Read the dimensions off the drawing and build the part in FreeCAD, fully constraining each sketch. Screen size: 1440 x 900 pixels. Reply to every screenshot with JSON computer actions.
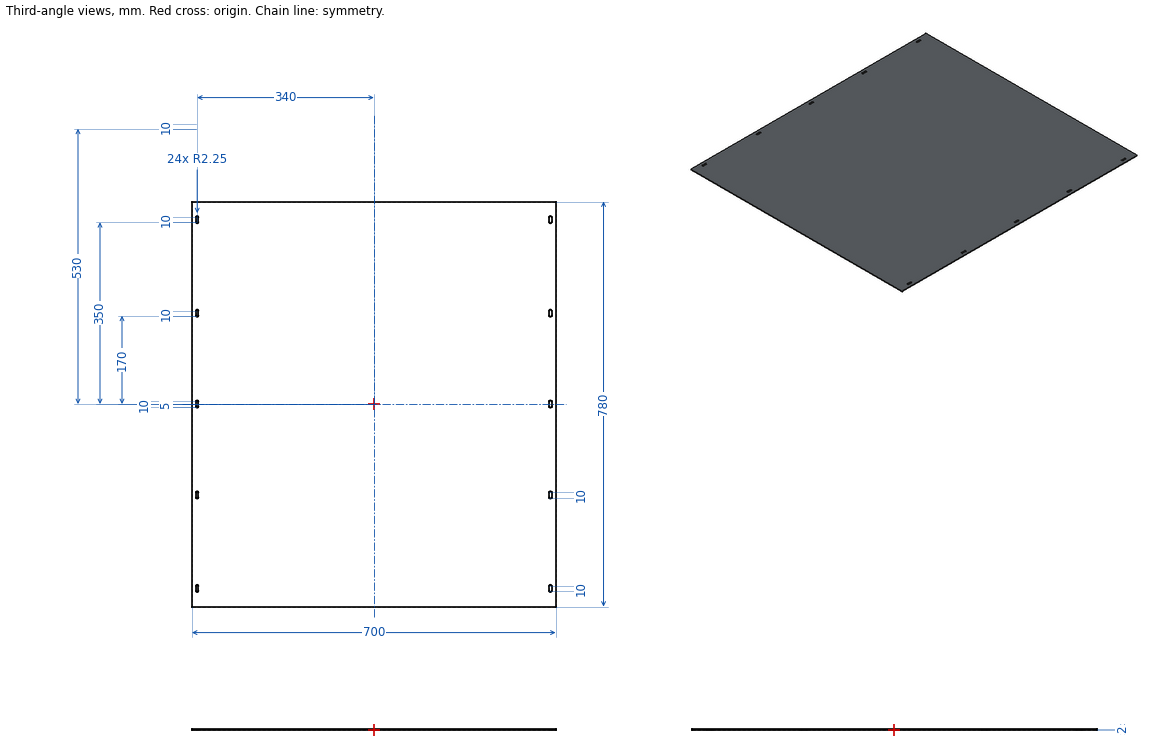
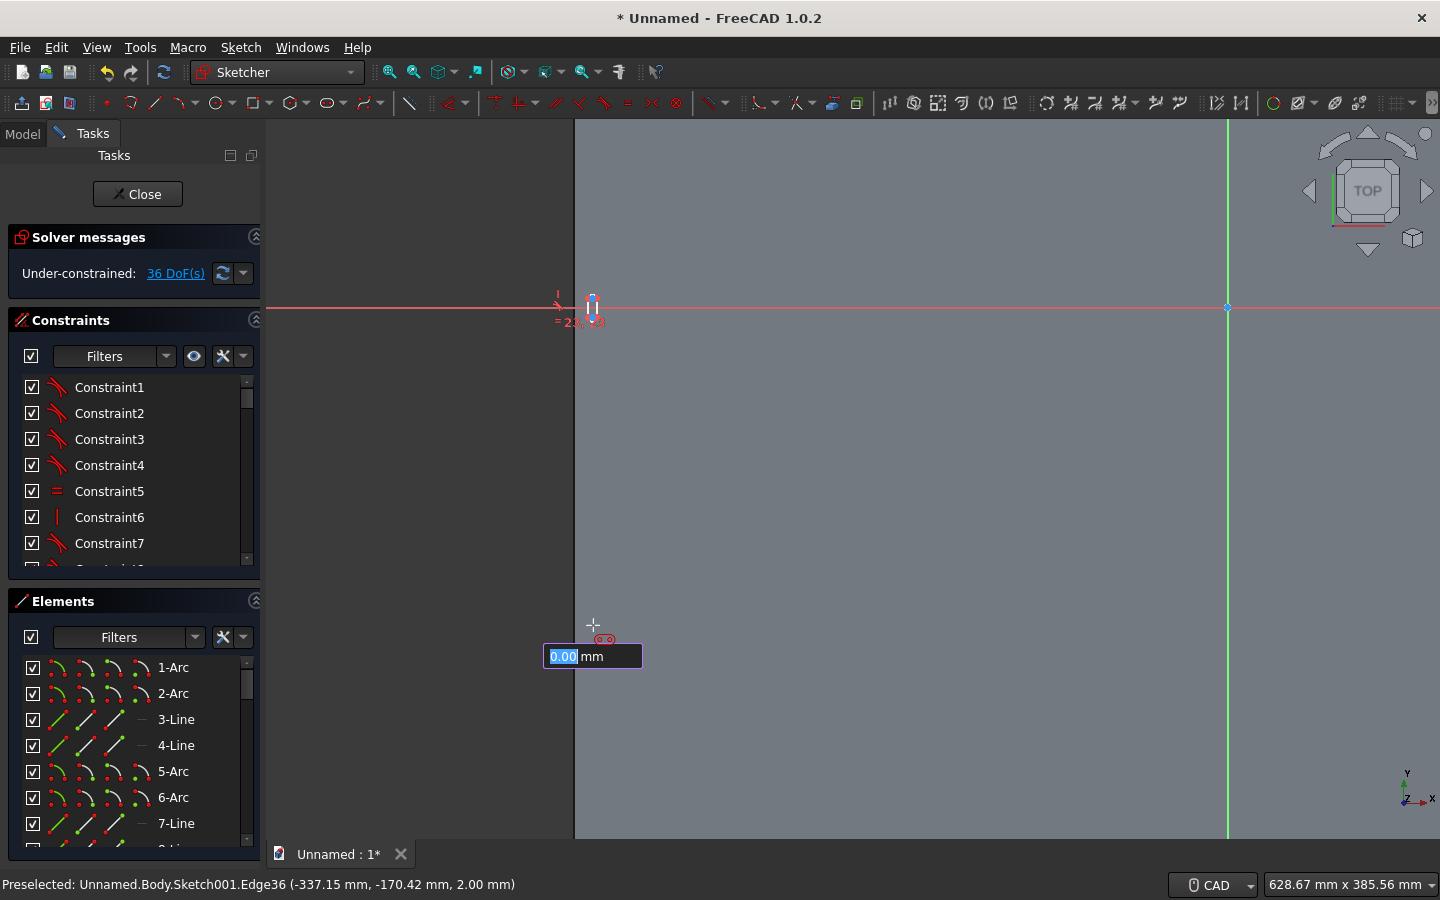
{"action": "scroll", "coordinate": [588, 634], "scroll_direction": "up", "scroll_amount": 7}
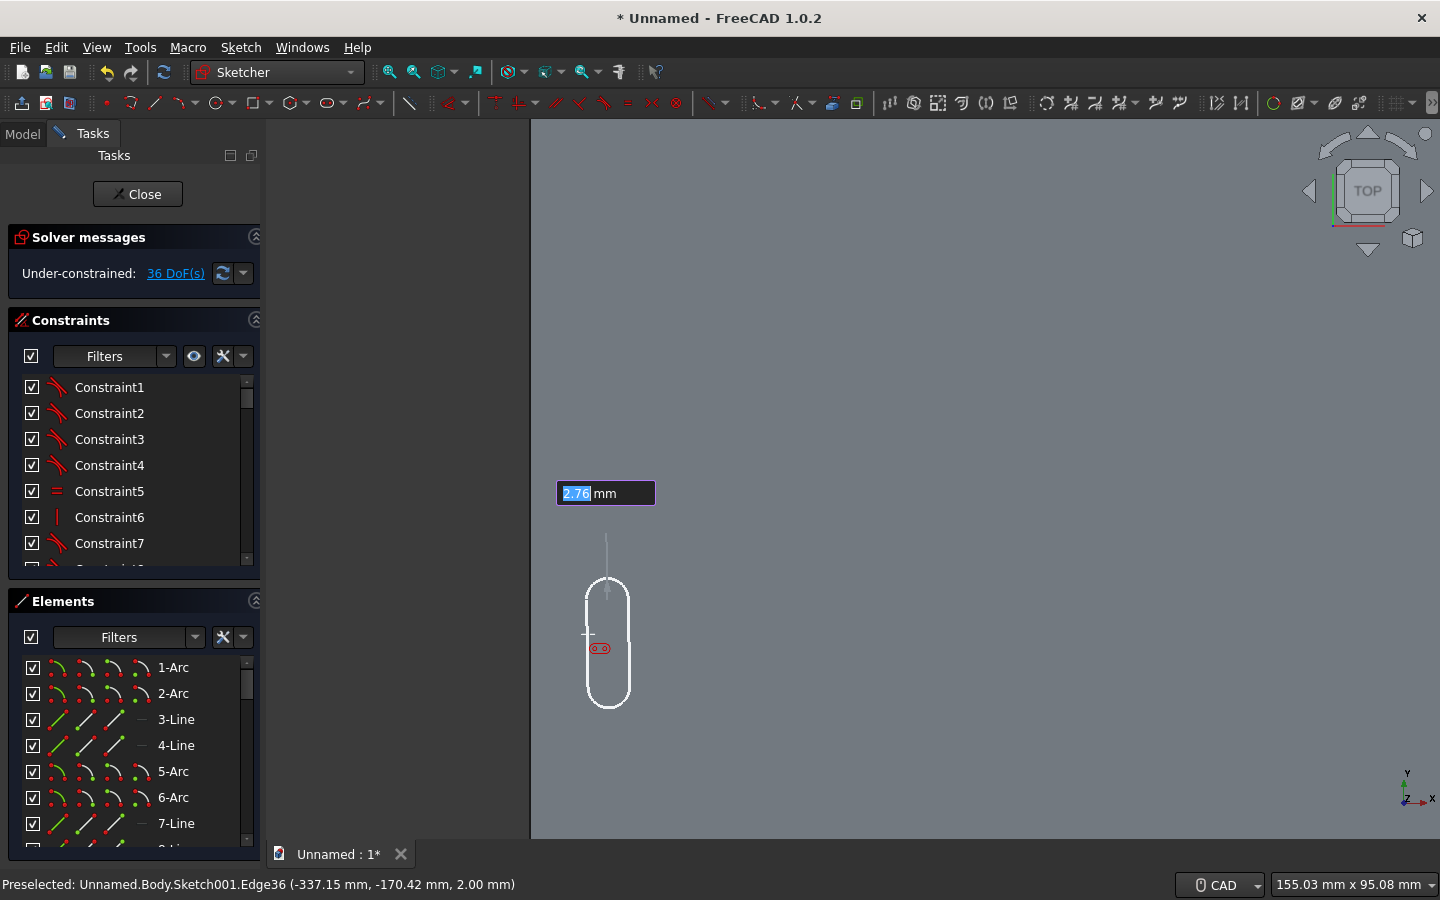
{"action": "left_click", "coordinate": [589, 633]}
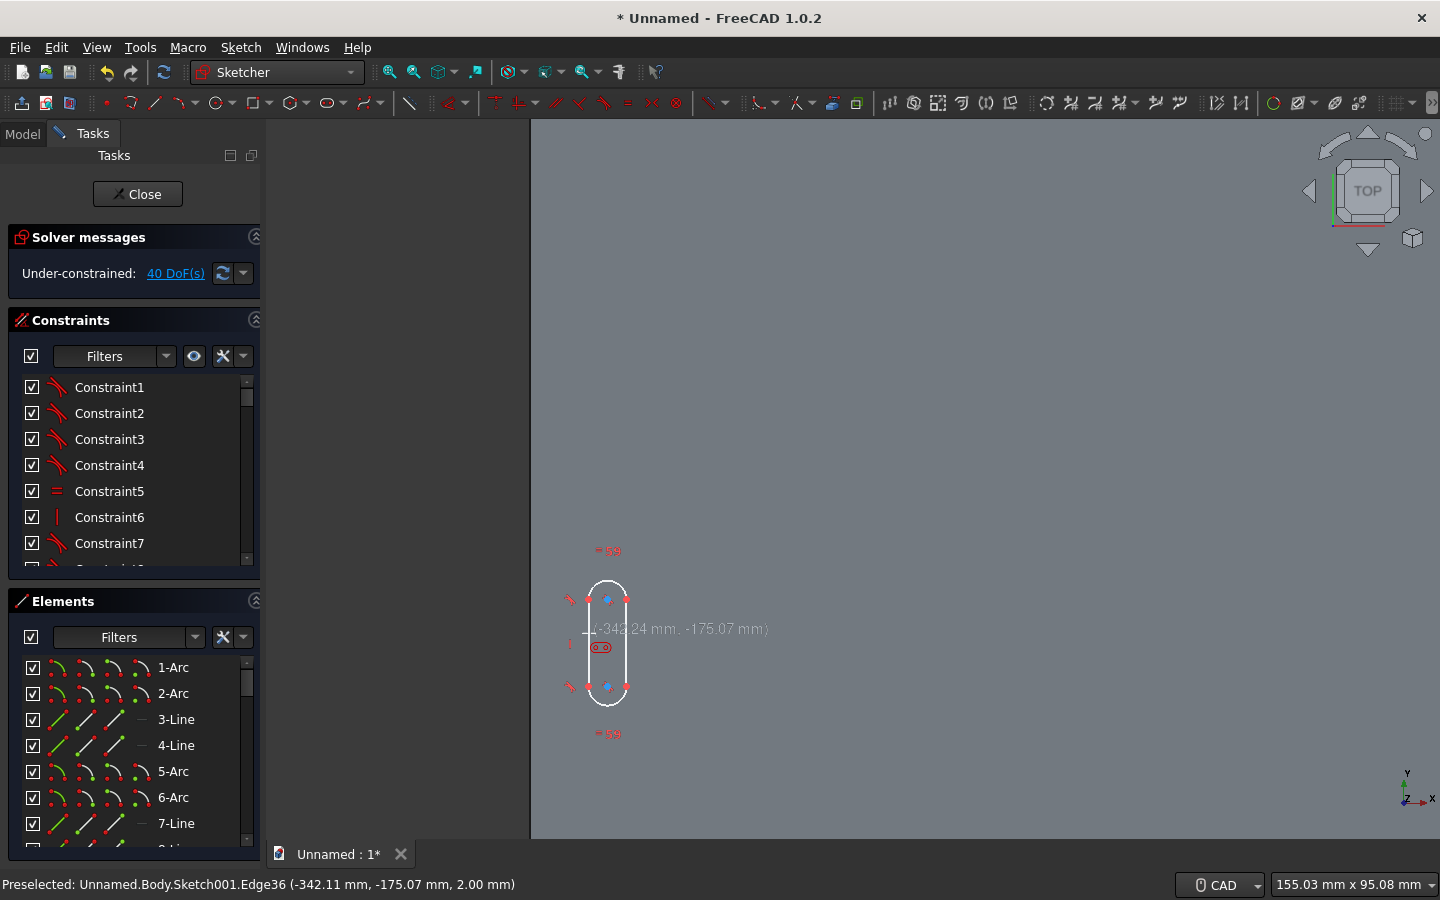
{"action": "scroll", "coordinate": [592, 628], "scroll_direction": "down", "scroll_amount": 13}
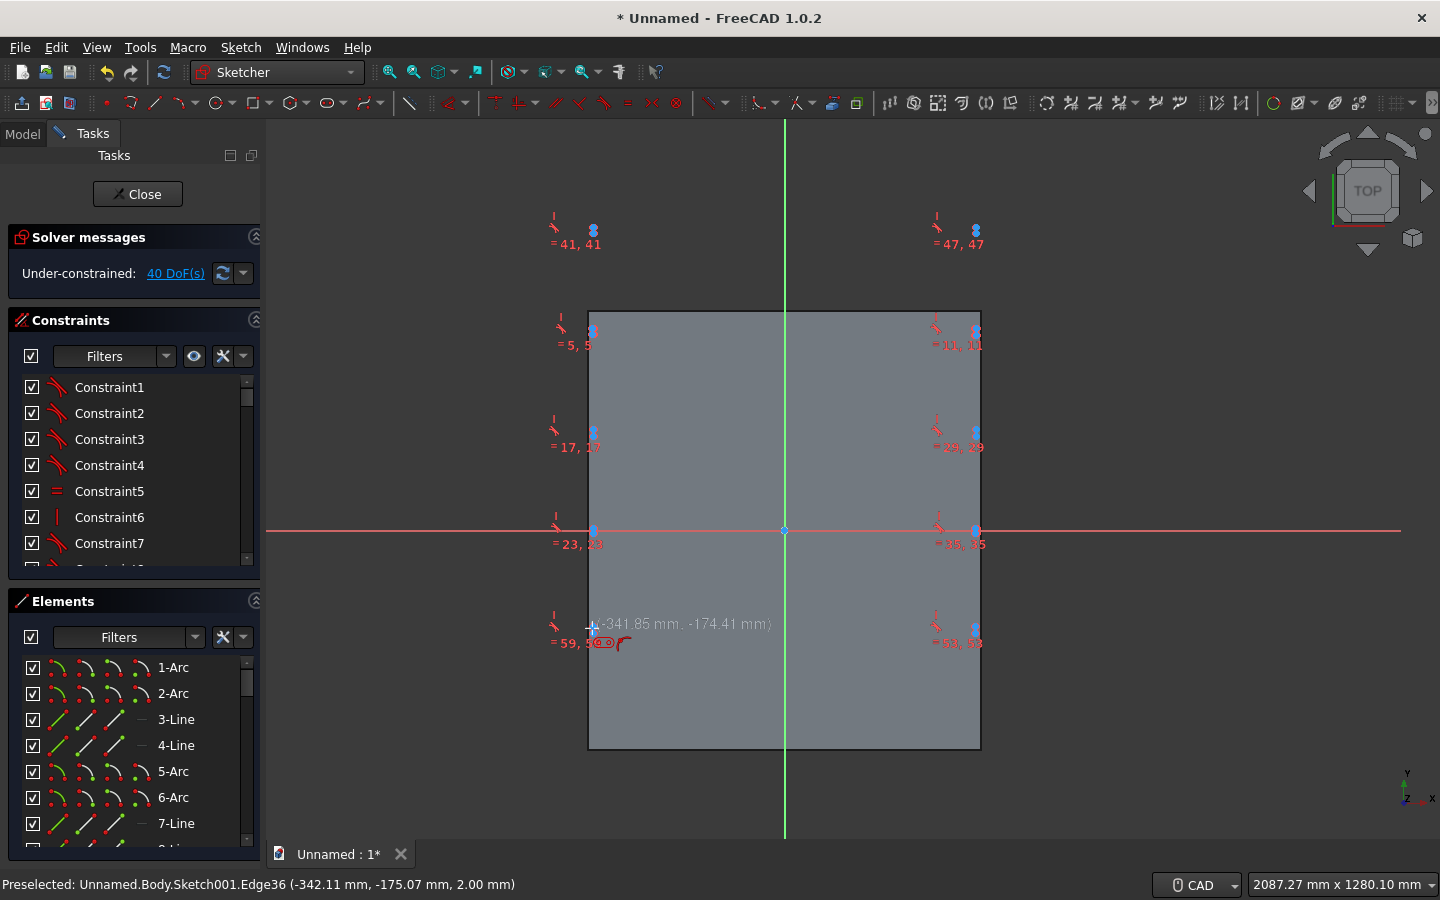
{"action": "scroll", "coordinate": [976, 733], "scroll_direction": "up", "scroll_amount": 15}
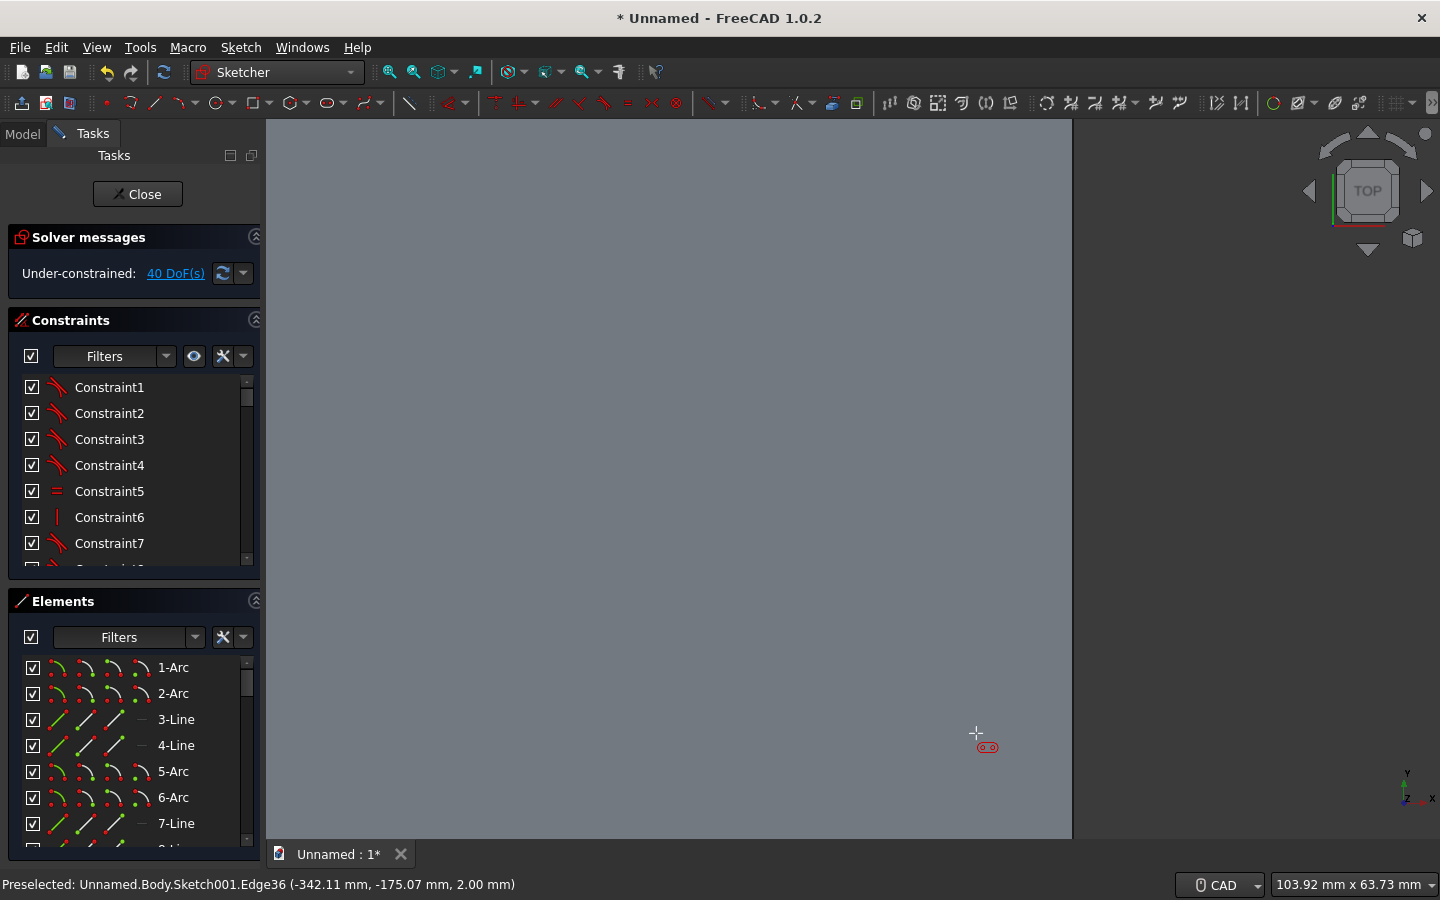
{"action": "scroll", "coordinate": [977, 733], "scroll_direction": "down", "scroll_amount": 15}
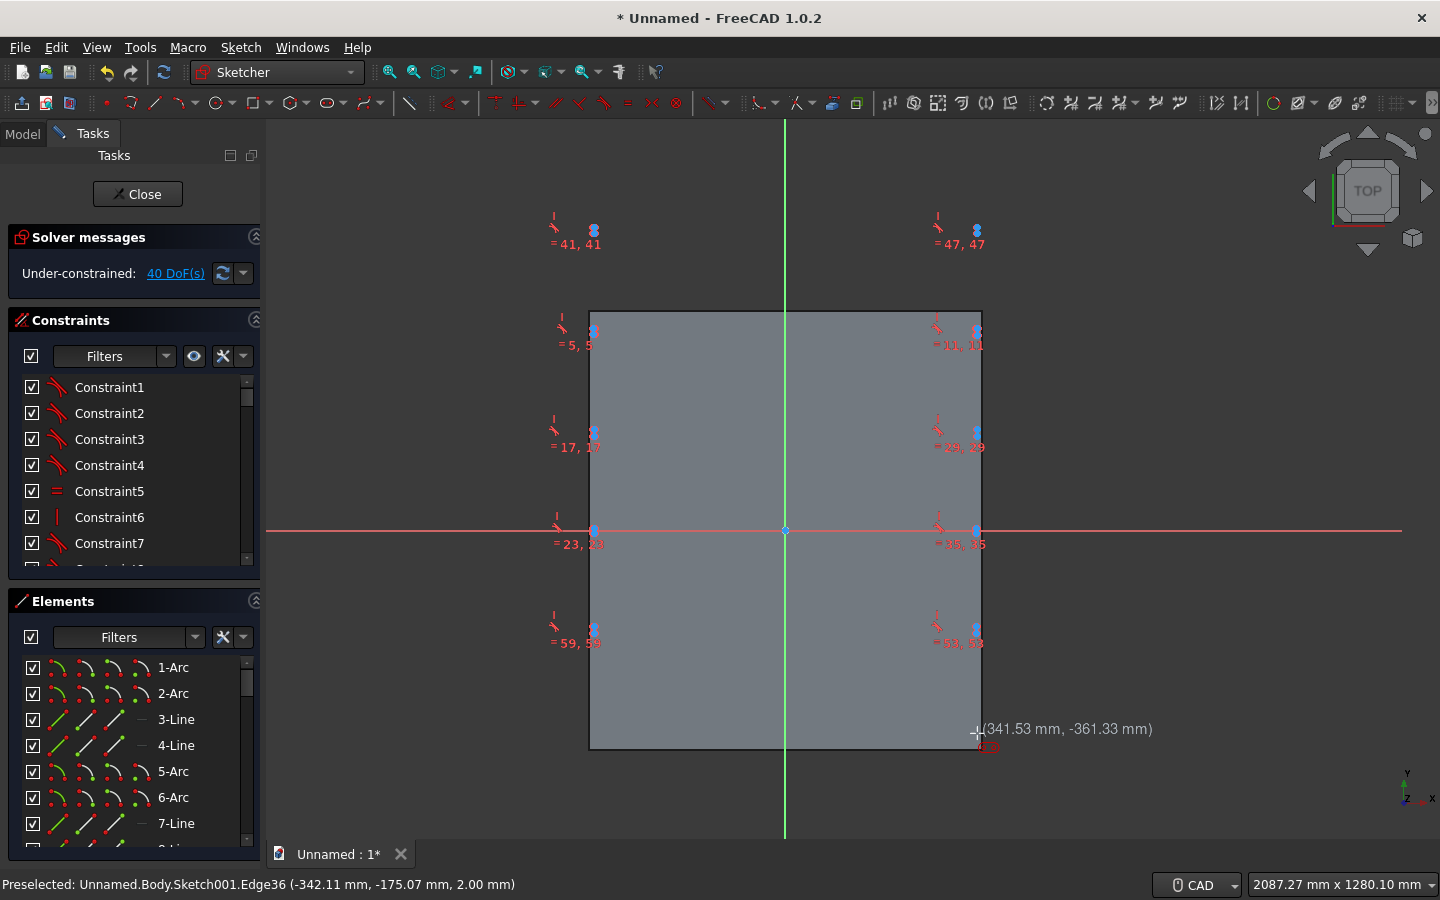
{"action": "left_click", "coordinate": [977, 733]}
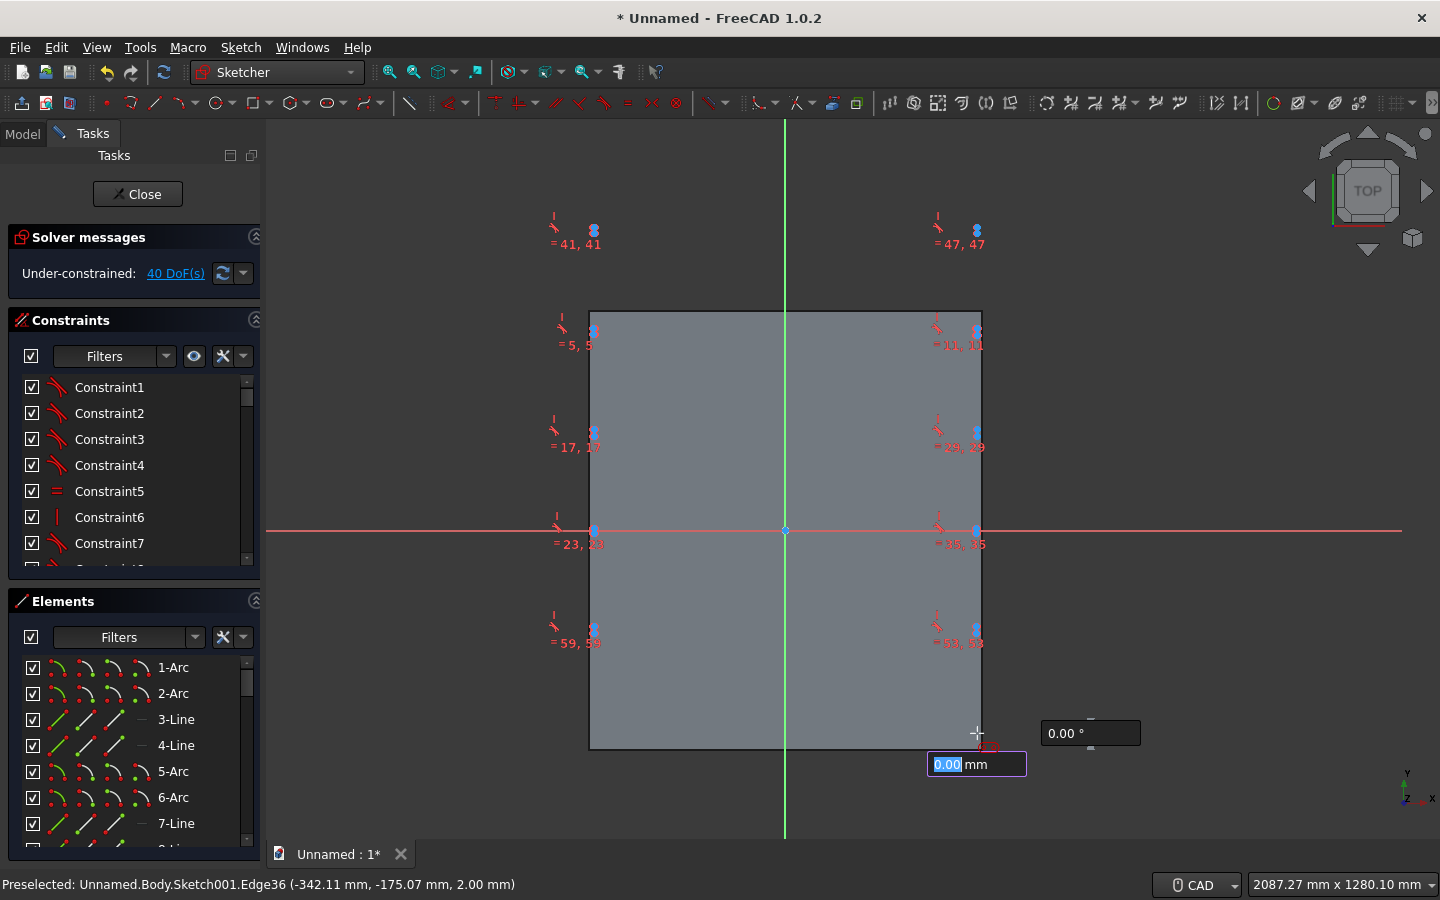
{"action": "scroll", "coordinate": [977, 727], "scroll_direction": "up", "scroll_amount": 6}